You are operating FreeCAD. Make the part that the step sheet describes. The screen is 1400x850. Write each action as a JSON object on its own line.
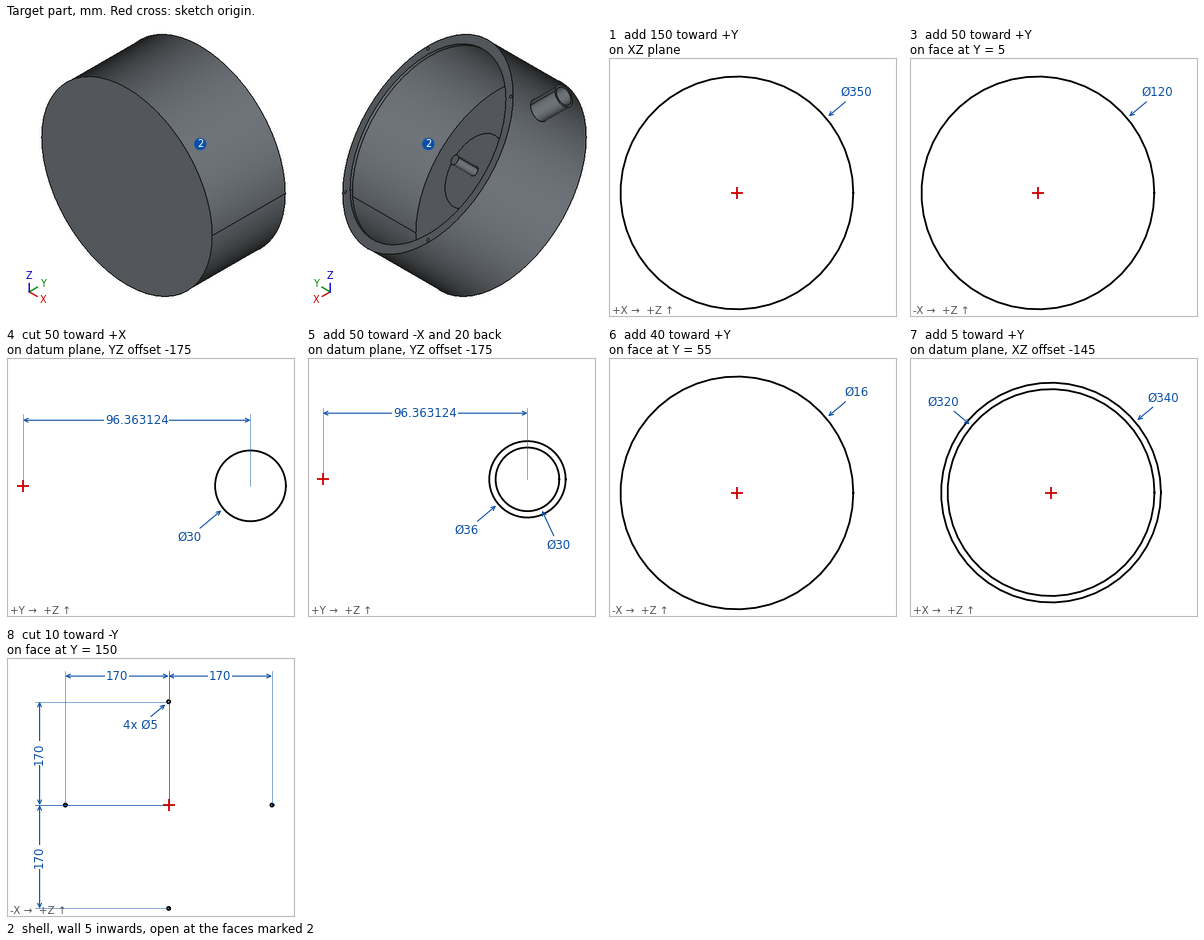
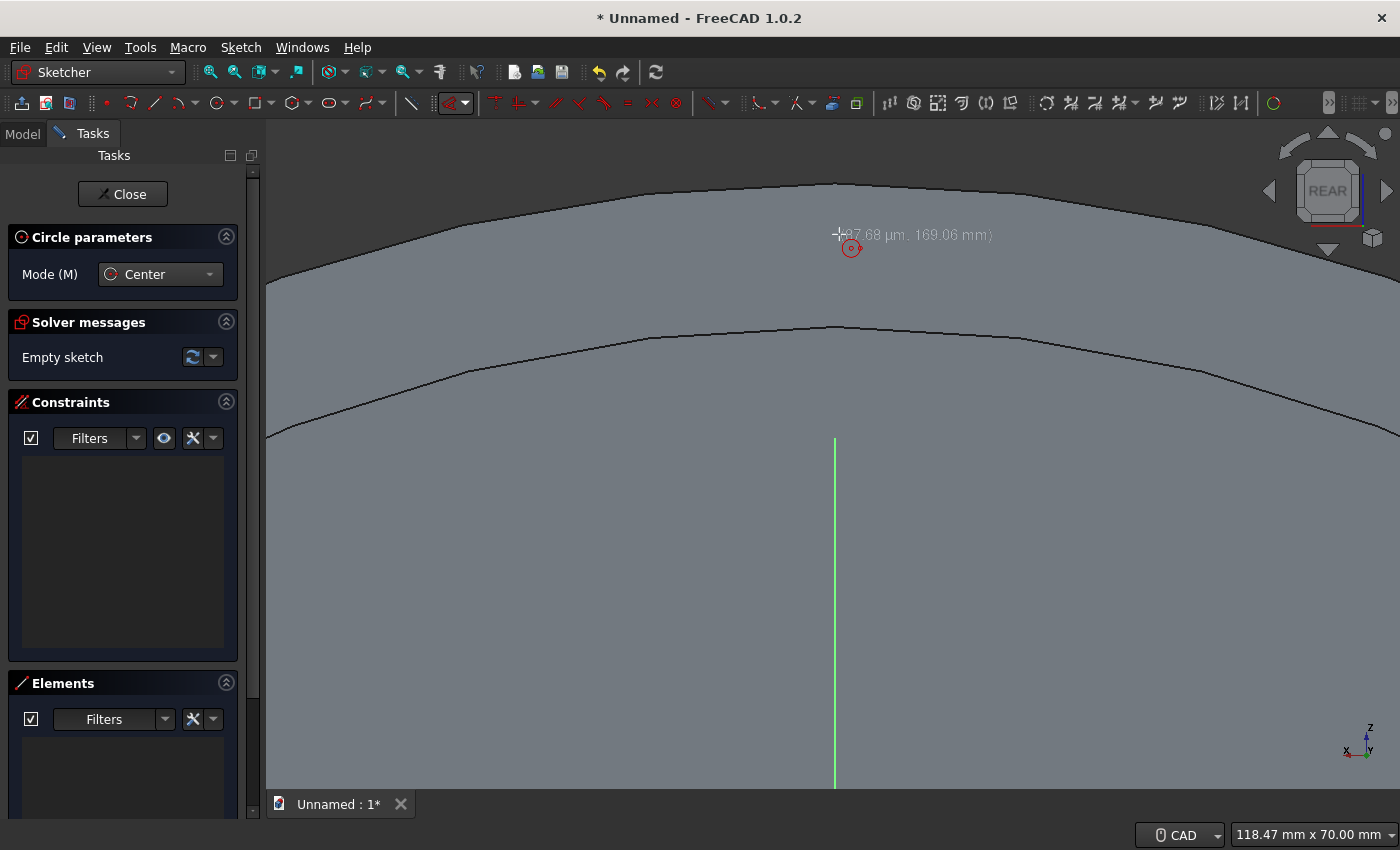
{"action": "scroll", "coordinate": [753, 234], "scroll_direction": "down", "scroll_amount": 10}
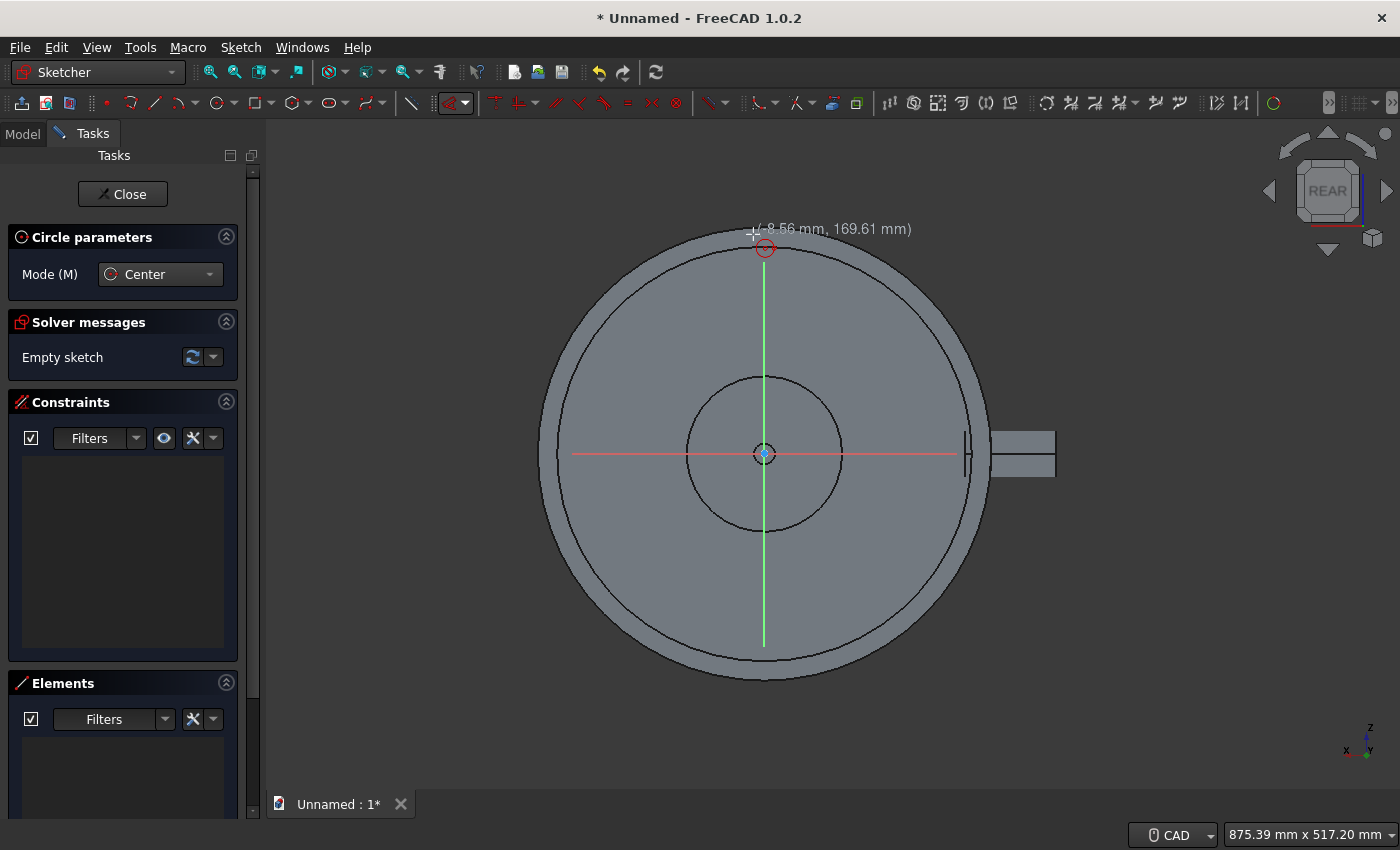
{"action": "left_click", "coordinate": [764, 234]}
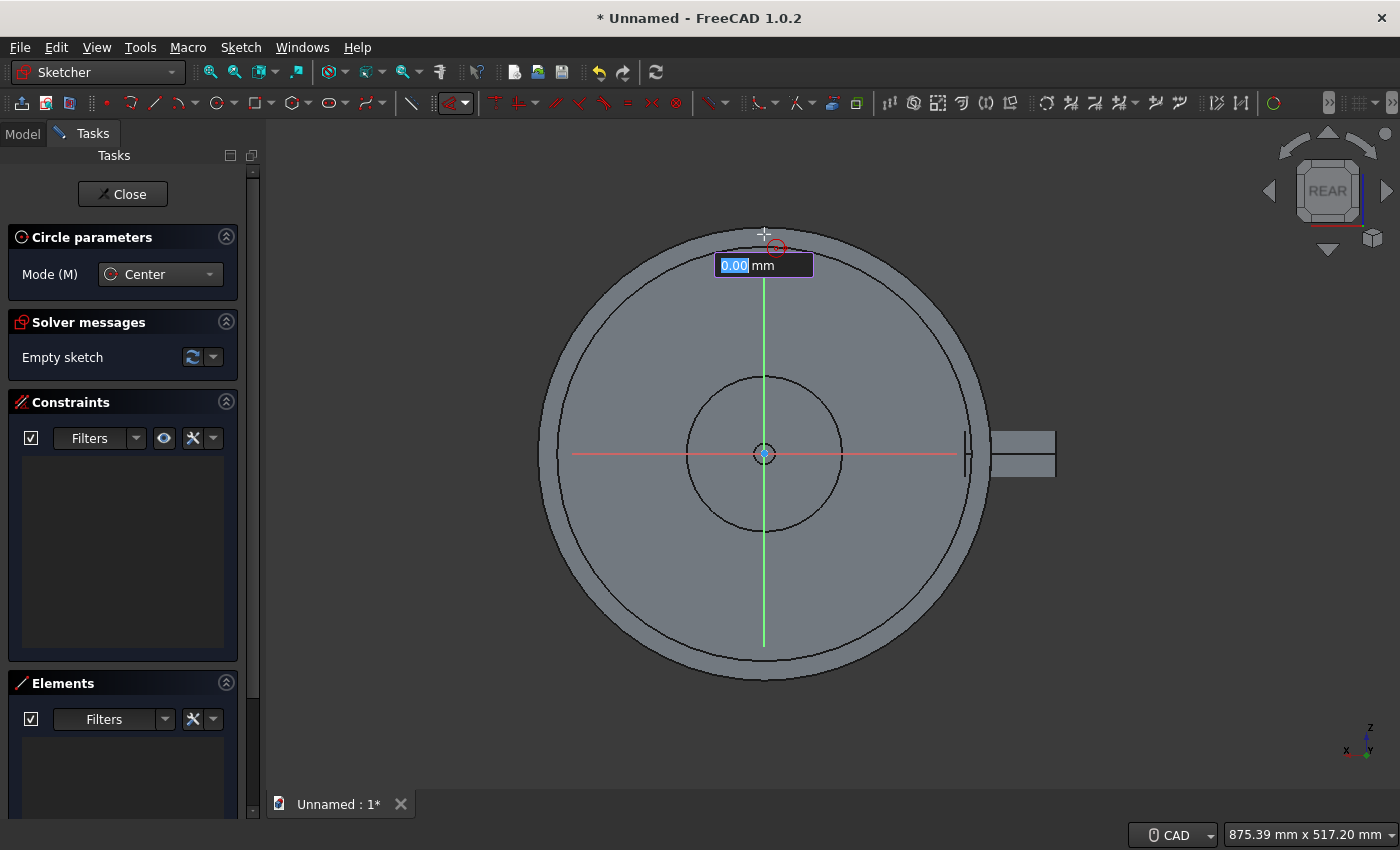
{"action": "scroll", "coordinate": [768, 233], "scroll_direction": "up", "scroll_amount": 9}
{"action": "mouse_move", "coordinate": [763, 230]}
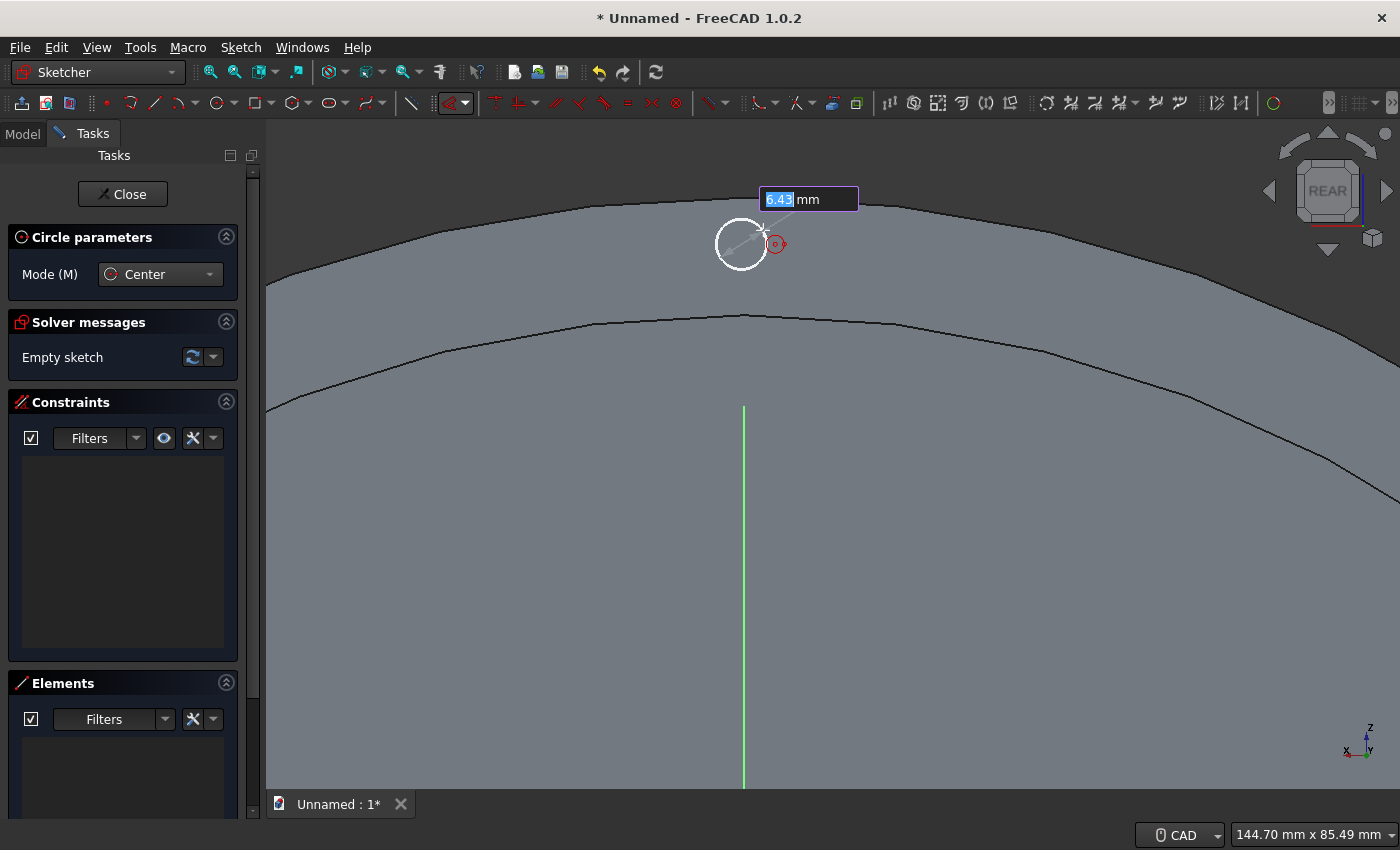
{"action": "type", "text": "5"}
{"action": "key", "text": "Return"}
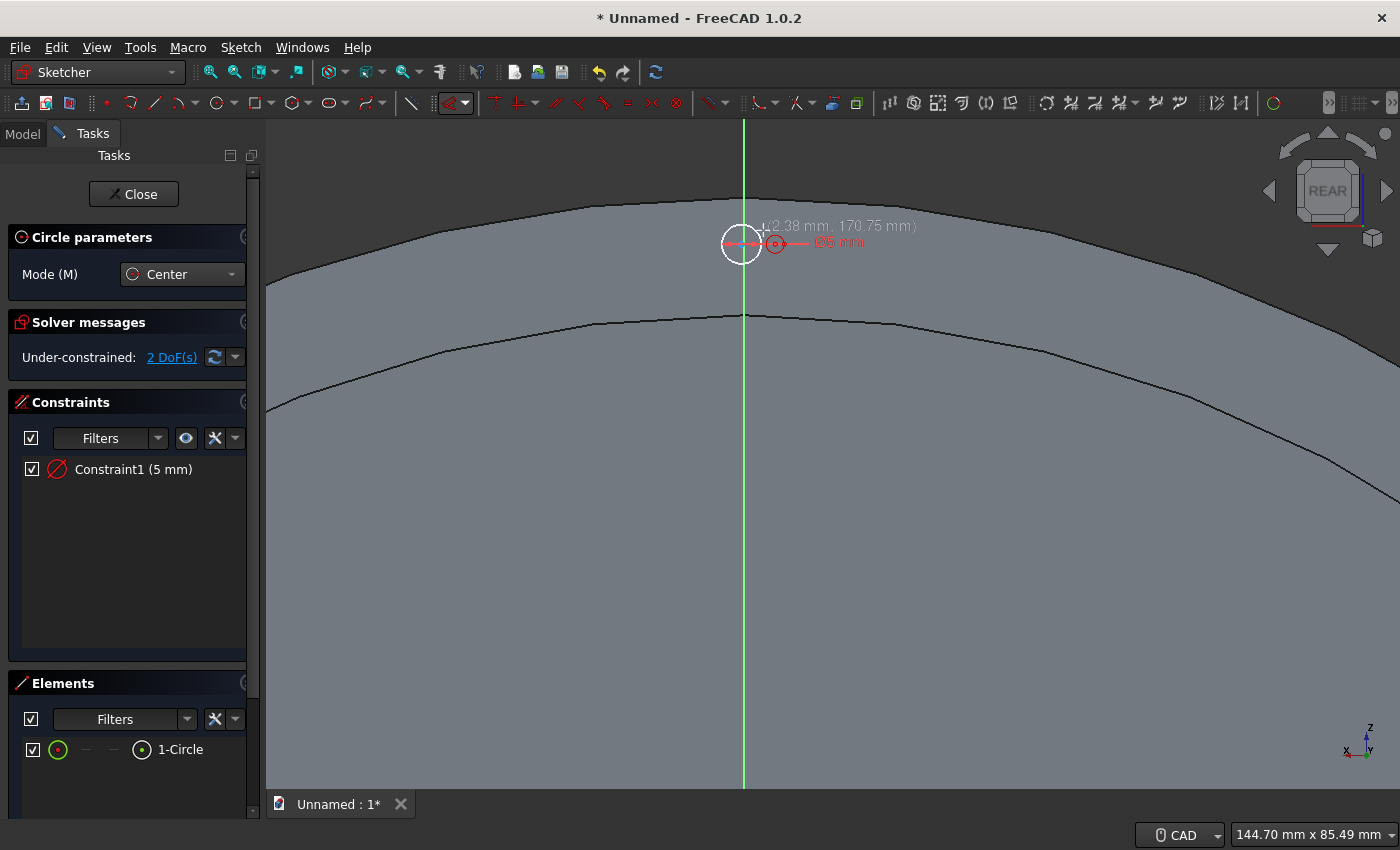
{"action": "scroll", "coordinate": [768, 233], "scroll_direction": "down", "scroll_amount": 9}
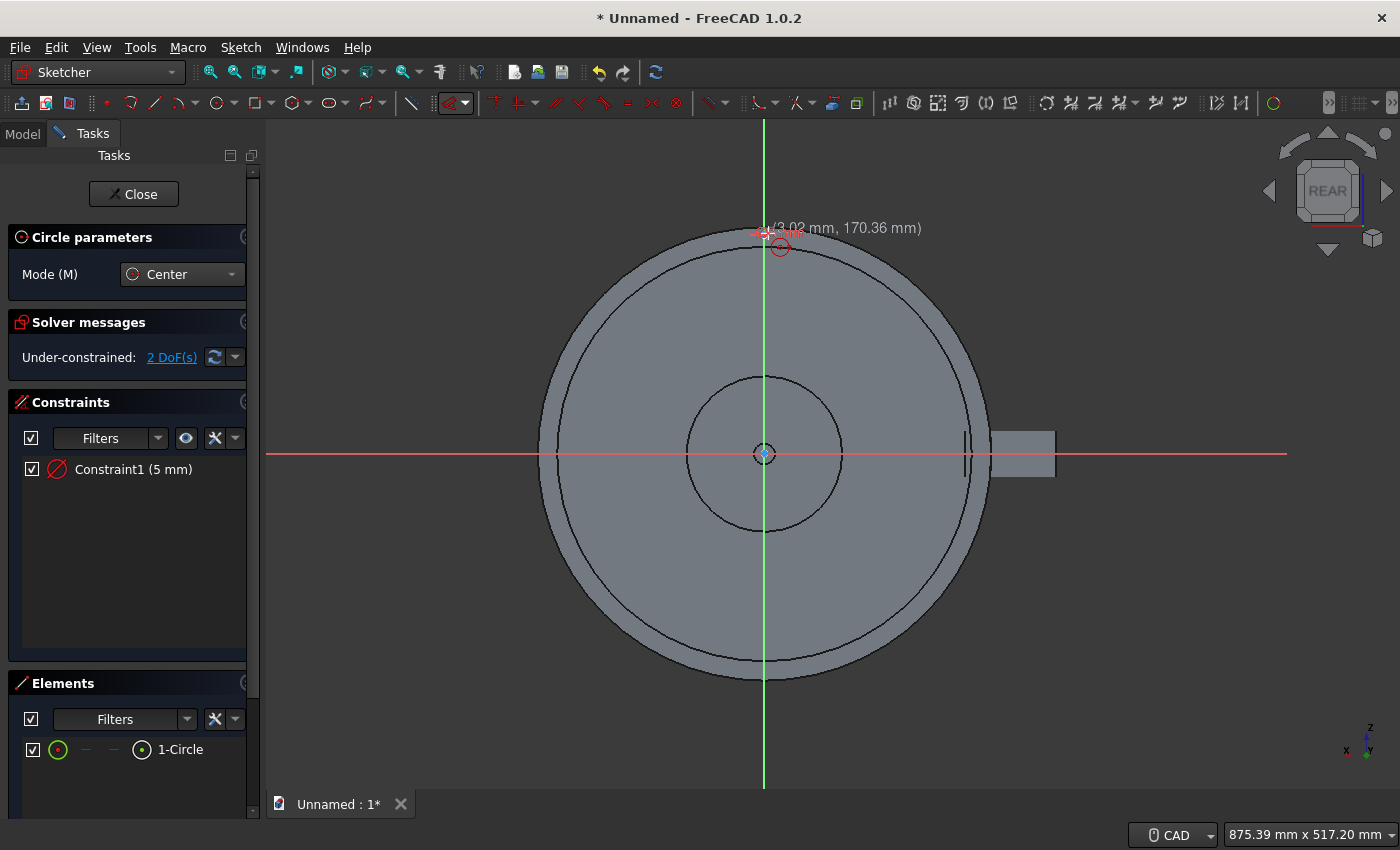
{"action": "scroll", "coordinate": [985, 454], "scroll_direction": "up", "scroll_amount": 10}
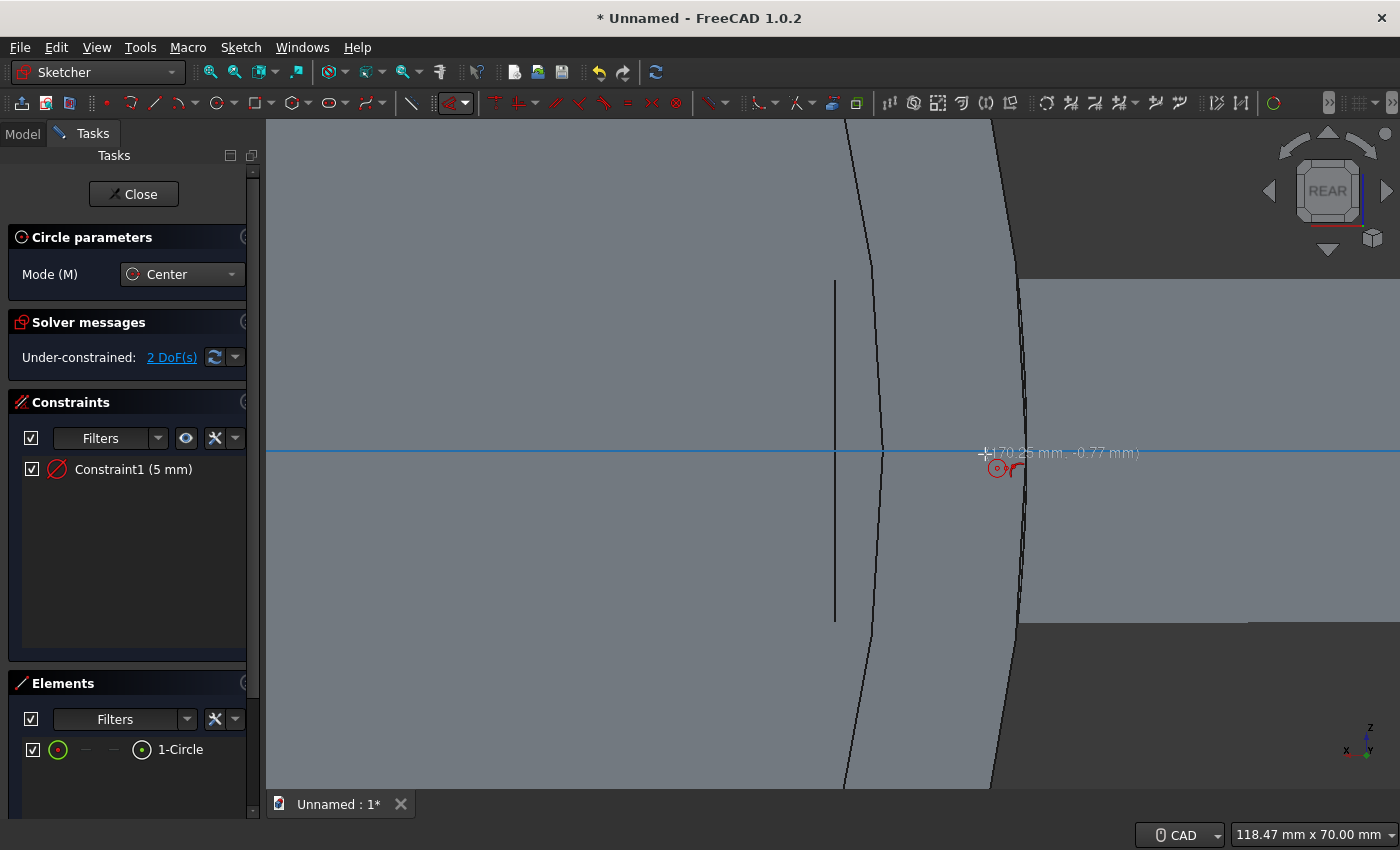
{"action": "scroll", "coordinate": [986, 455], "scroll_direction": "down", "scroll_amount": 10}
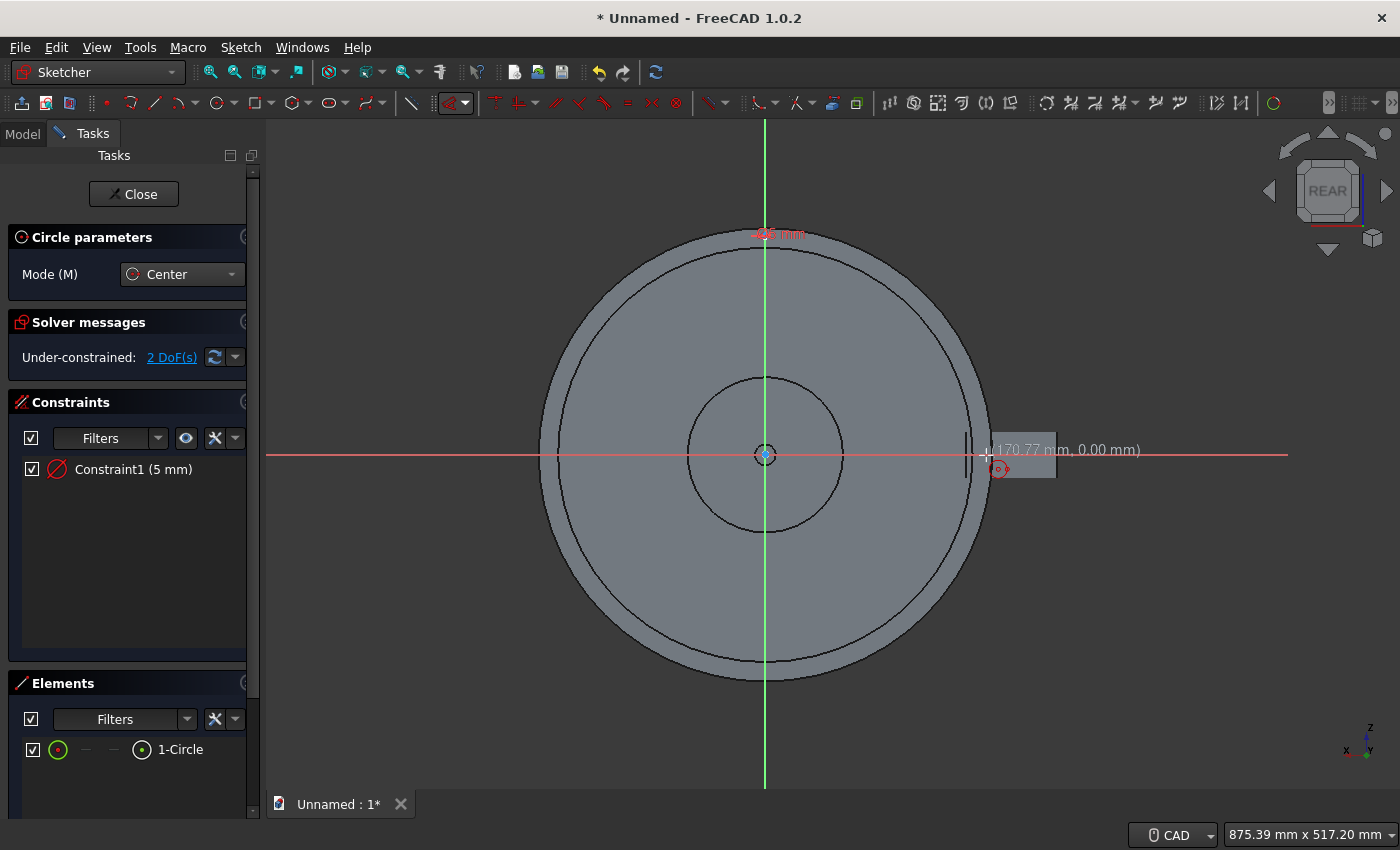
{"action": "left_click", "coordinate": [986, 455]}